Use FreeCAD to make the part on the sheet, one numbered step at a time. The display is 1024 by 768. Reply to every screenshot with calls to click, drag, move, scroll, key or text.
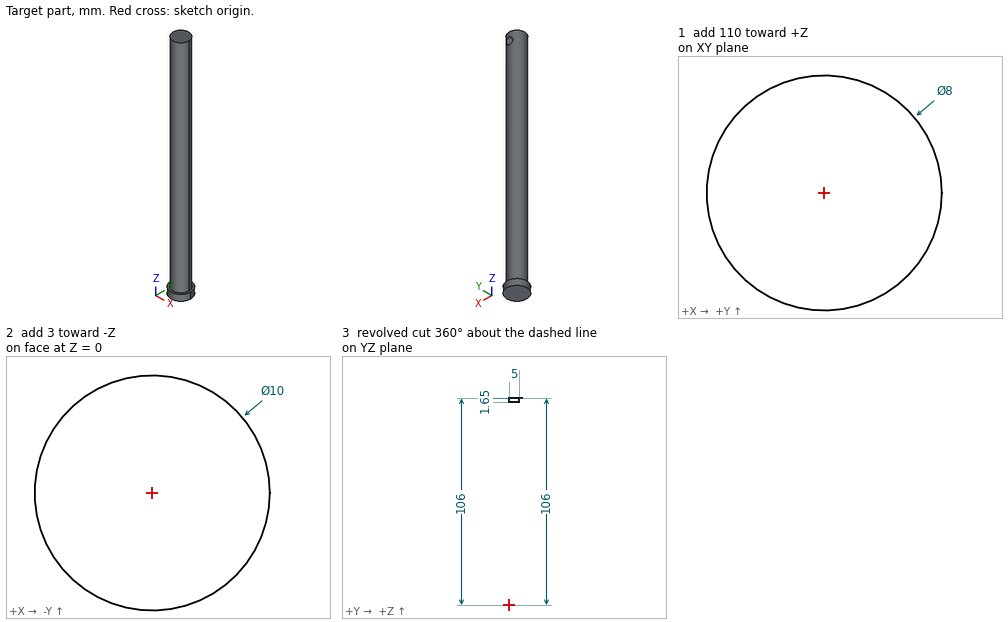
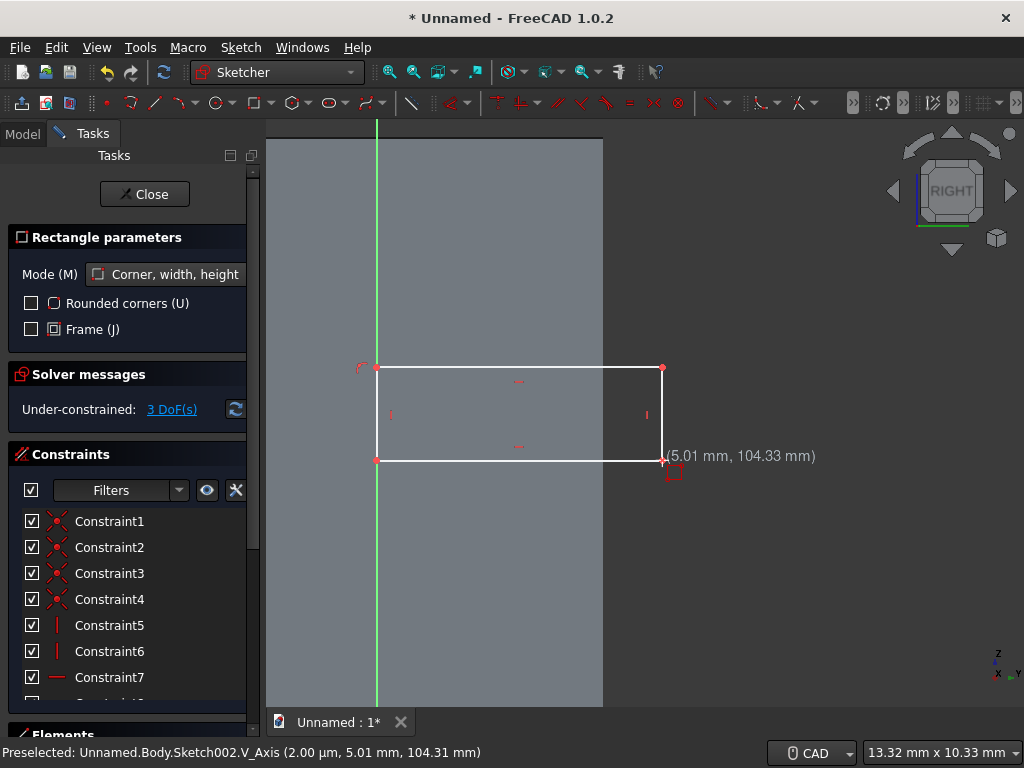
click(156, 104)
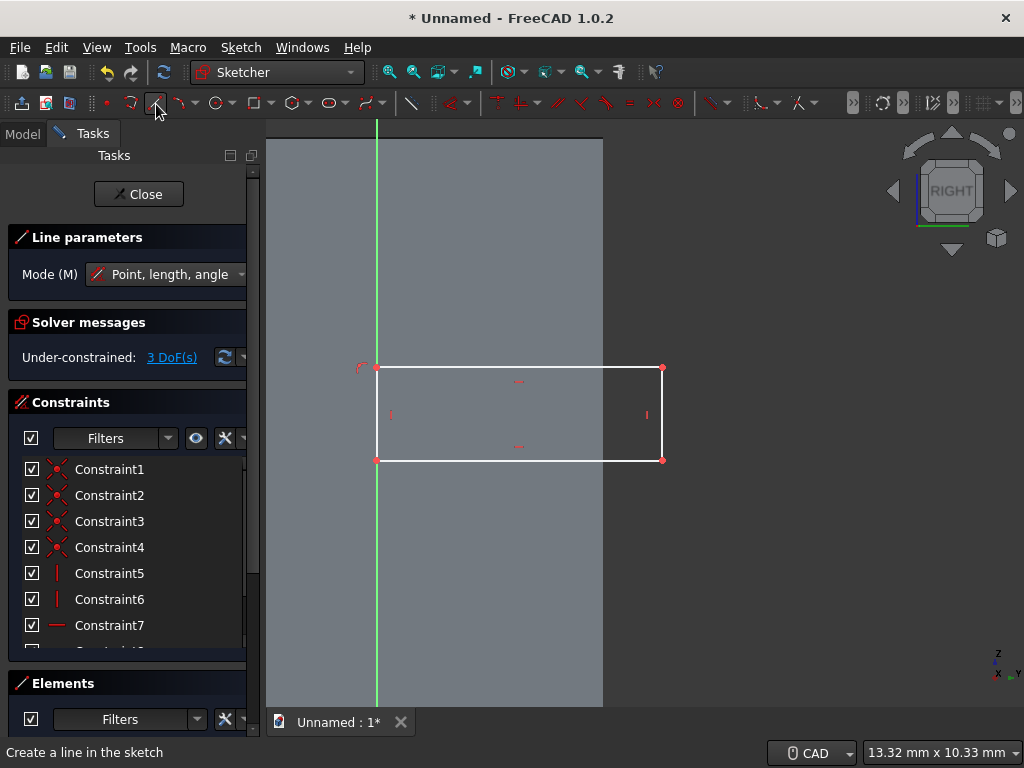
click(690, 366)
click(775, 366)
key(Escape)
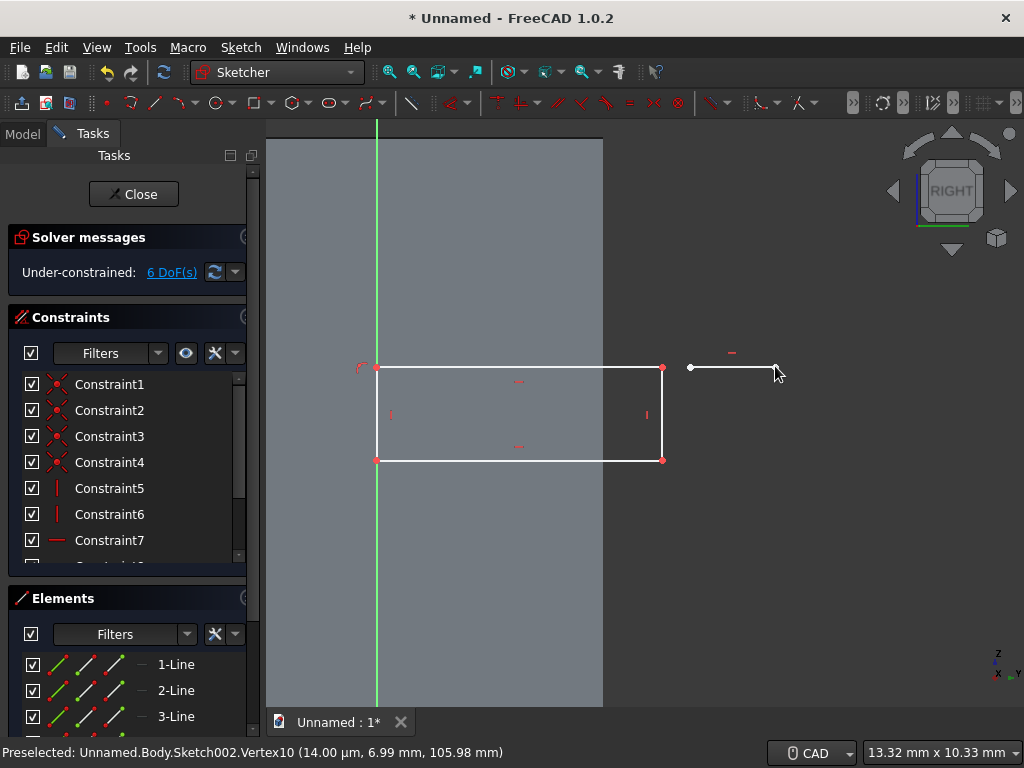
click(716, 367)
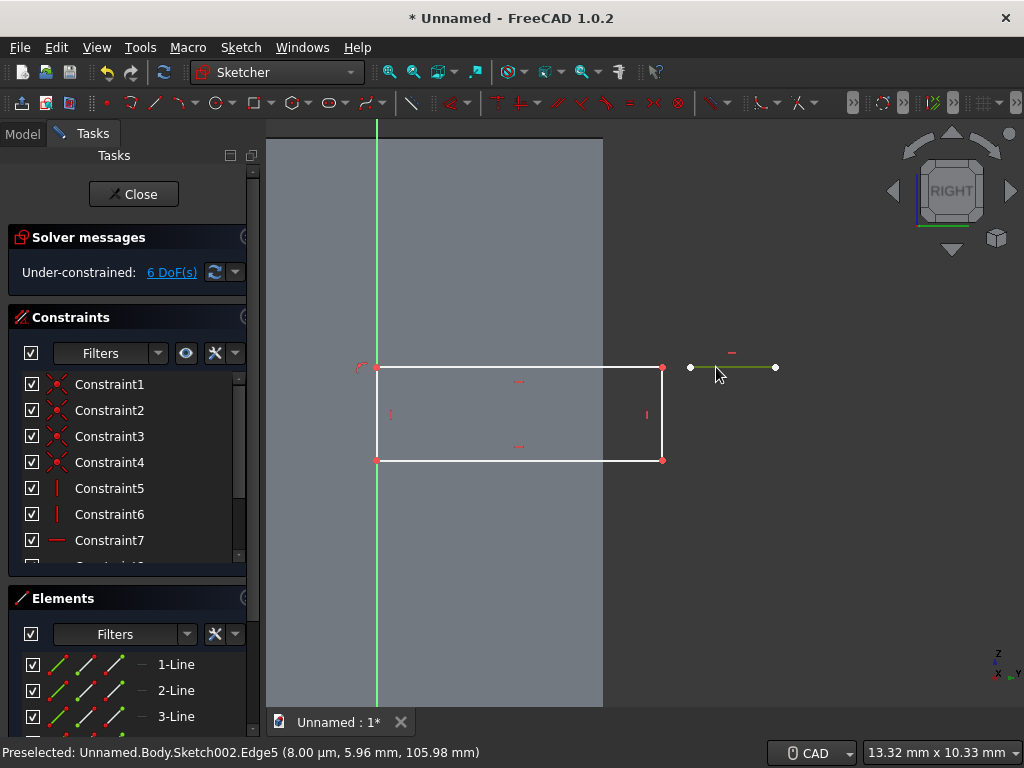
click(412, 104)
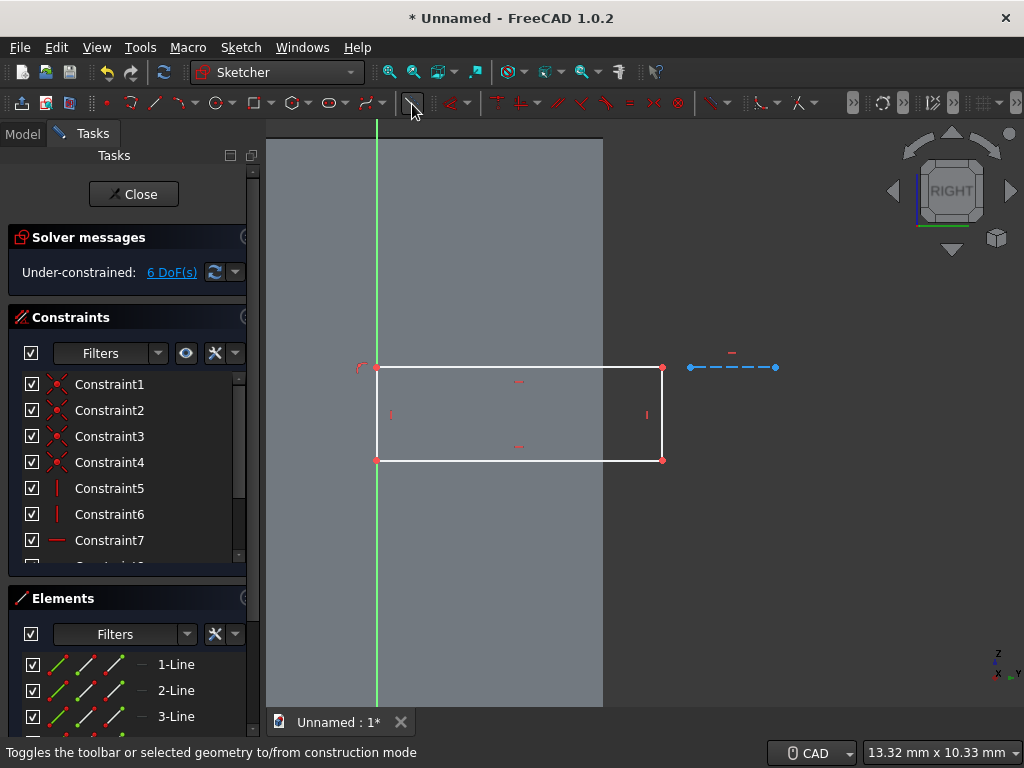
click(450, 104)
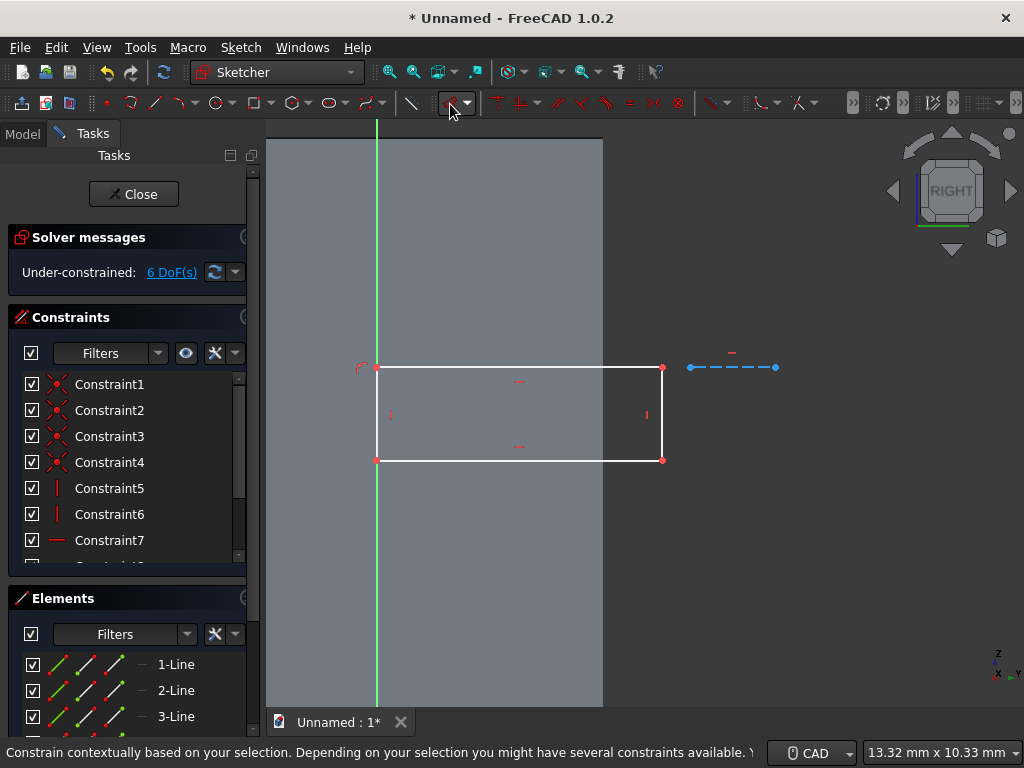
click(462, 461)
click(519, 495)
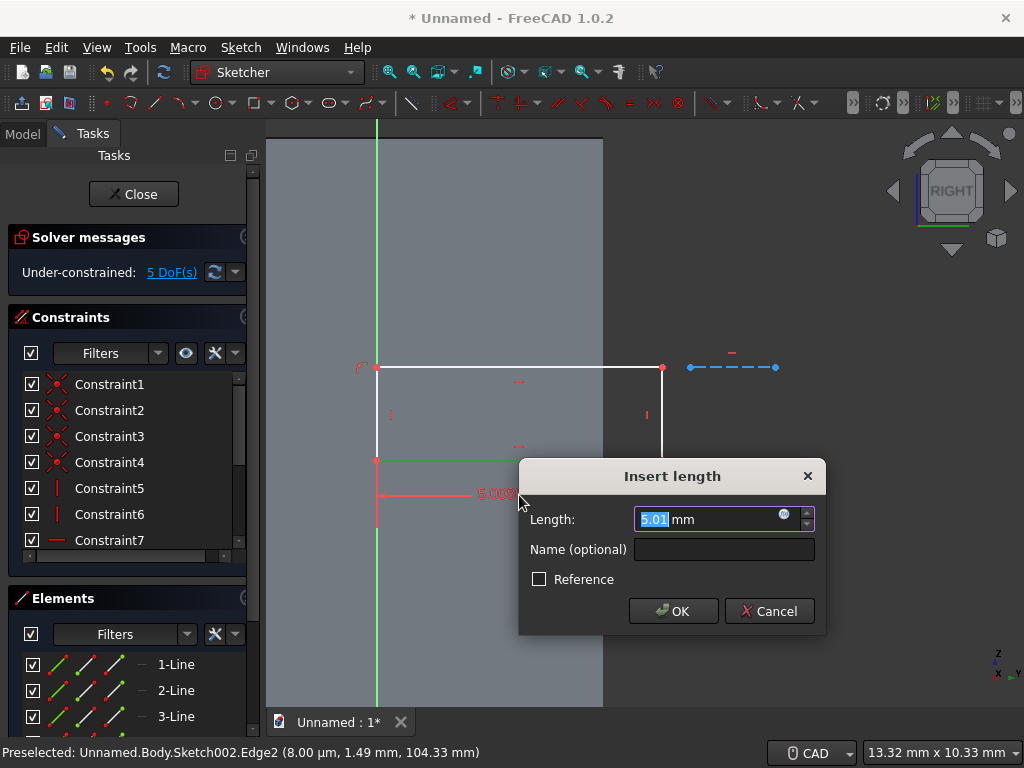
text(5)
key(Return)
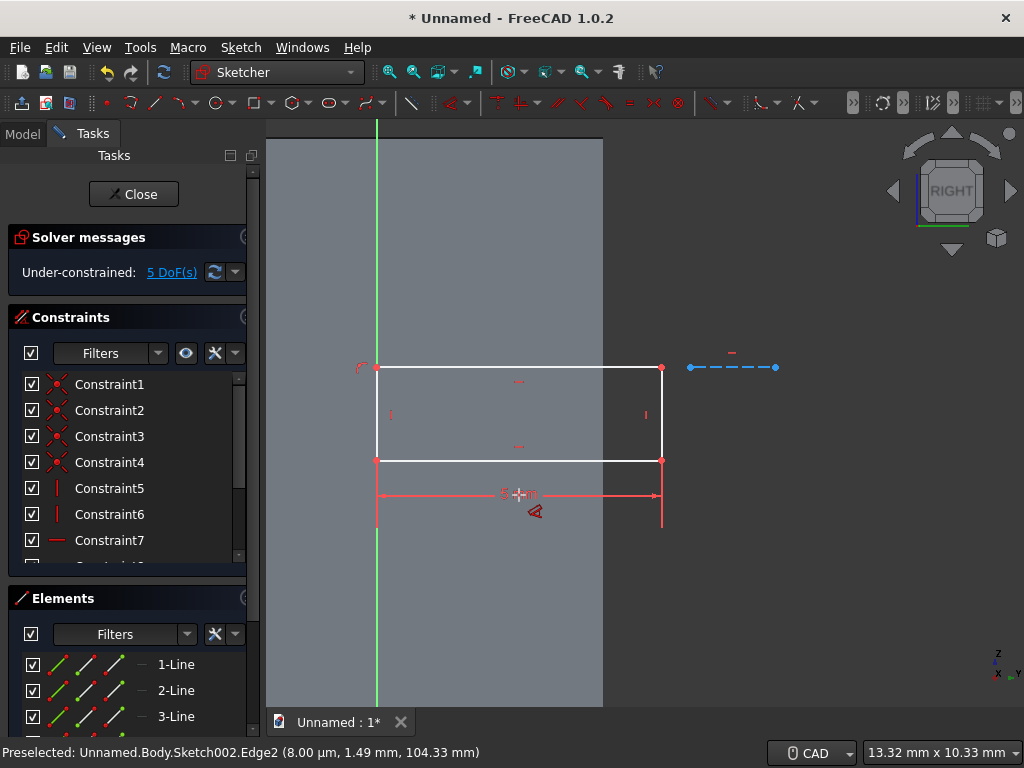
click(377, 395)
click(343, 414)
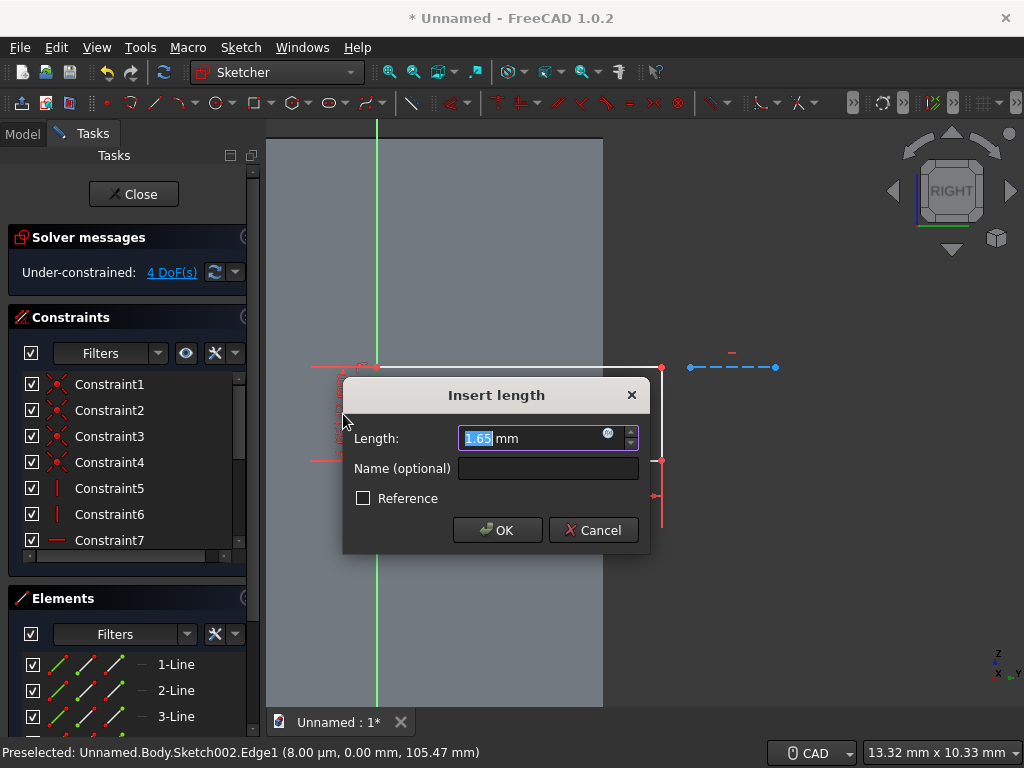
text(1.65)
key(Return)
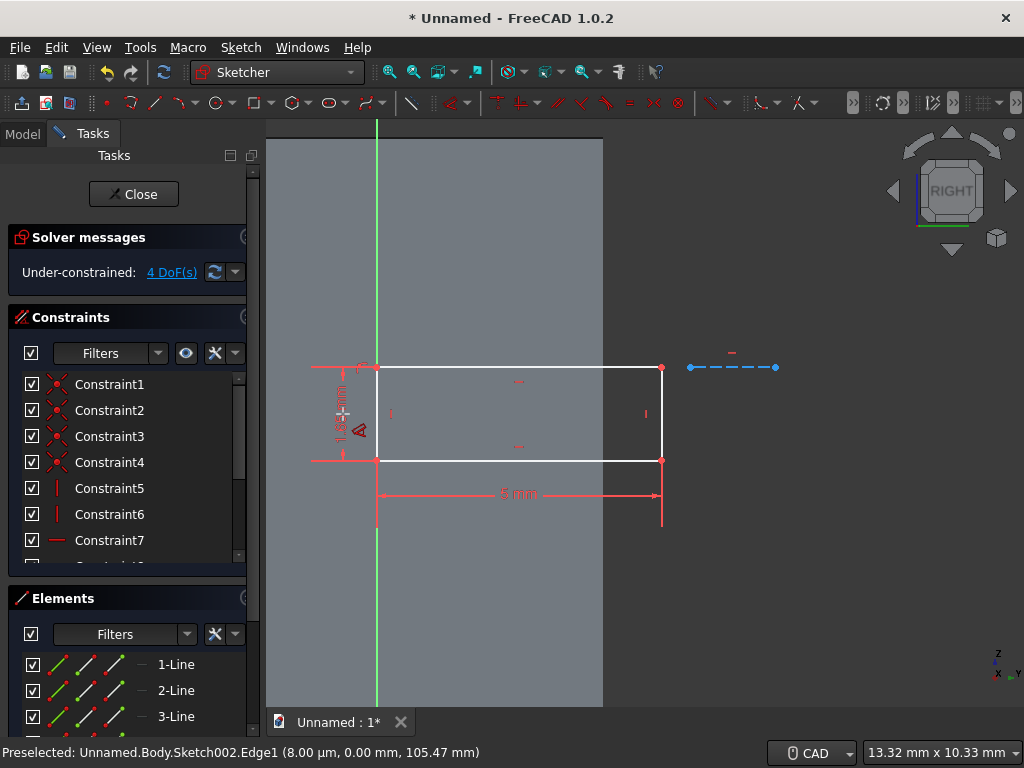
click(377, 367)
click(343, 523)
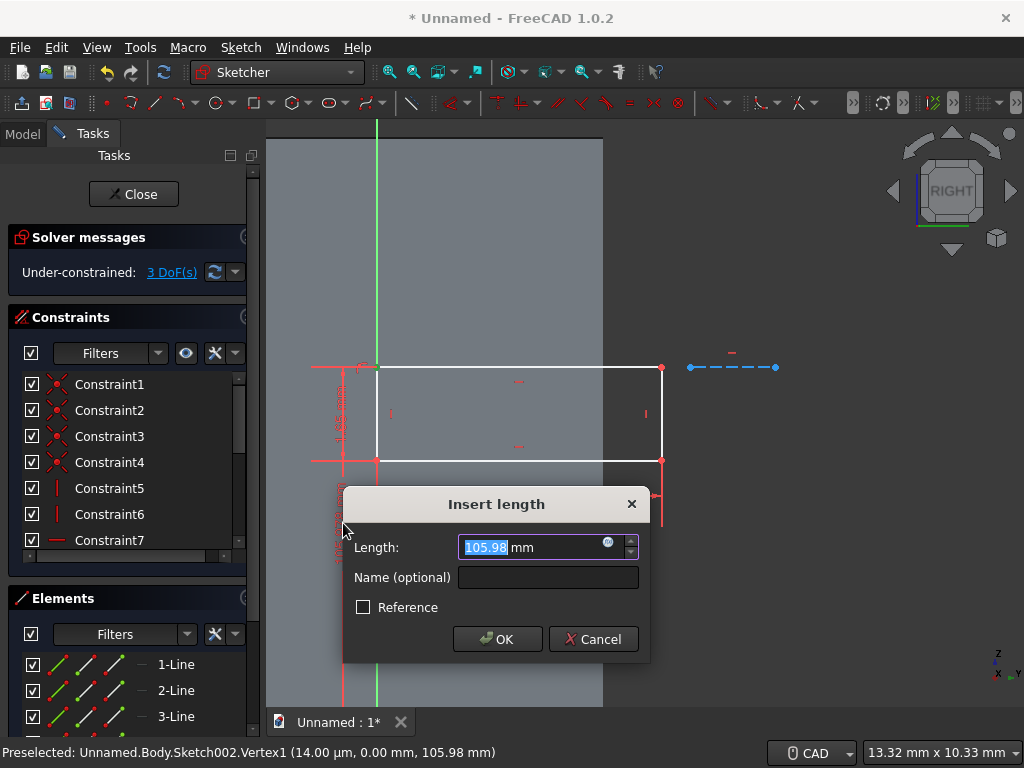
text(106)
key(Return)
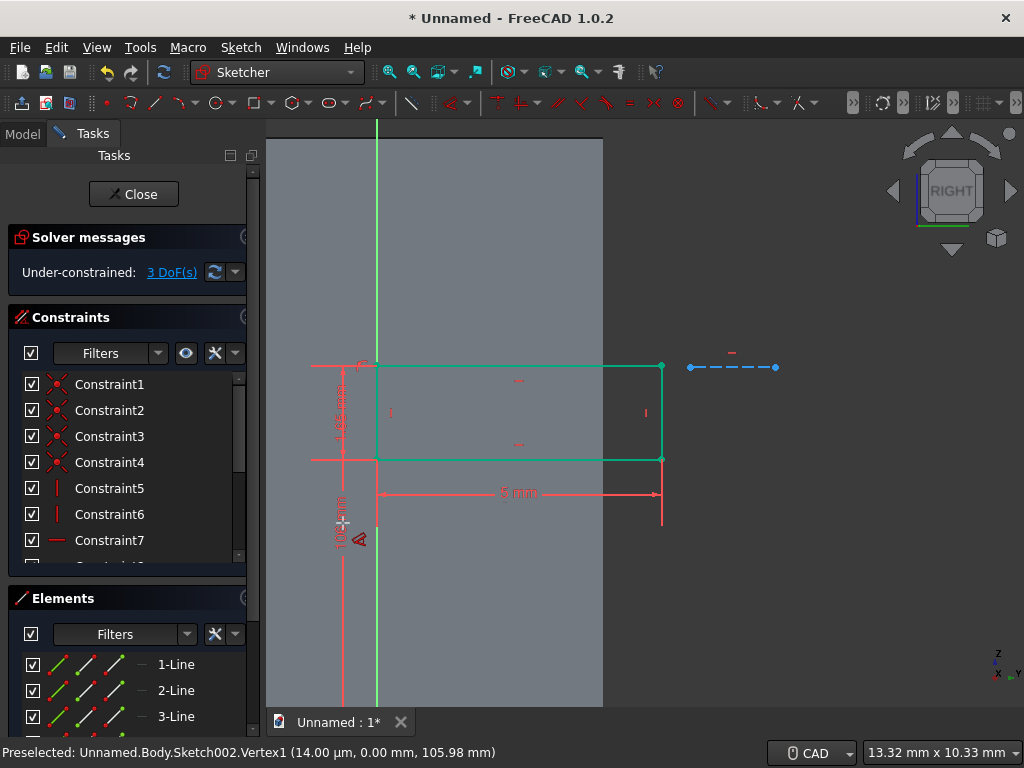
click(690, 367)
click(343, 451)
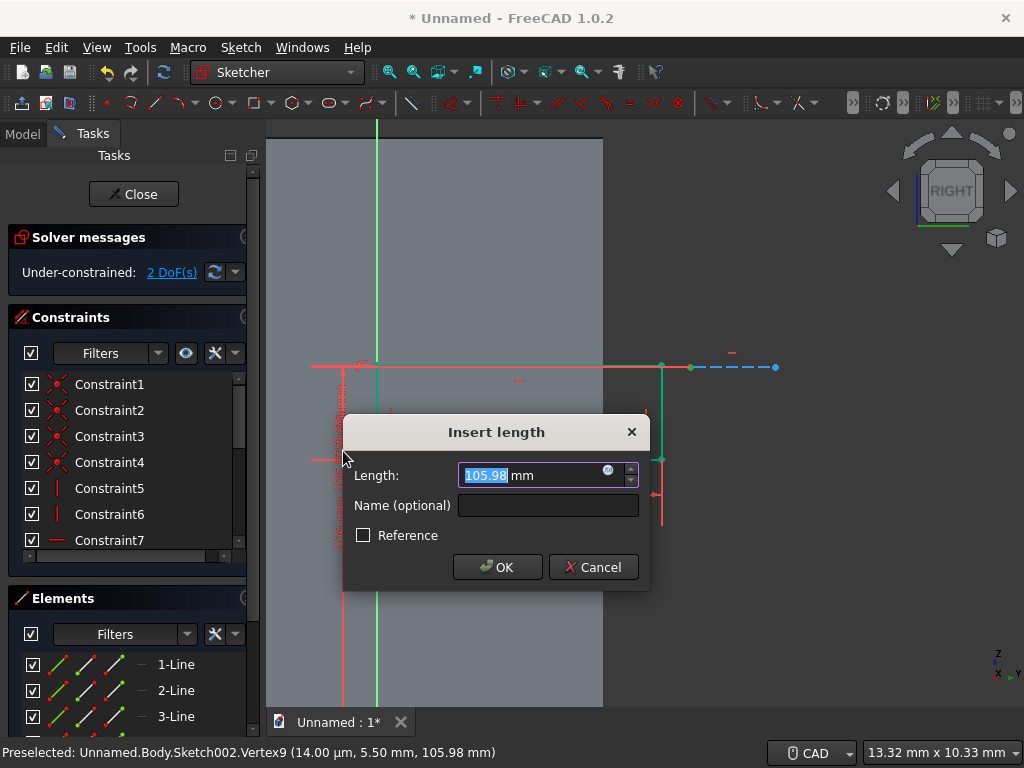
text(106)
key(Return)
key(Escape)